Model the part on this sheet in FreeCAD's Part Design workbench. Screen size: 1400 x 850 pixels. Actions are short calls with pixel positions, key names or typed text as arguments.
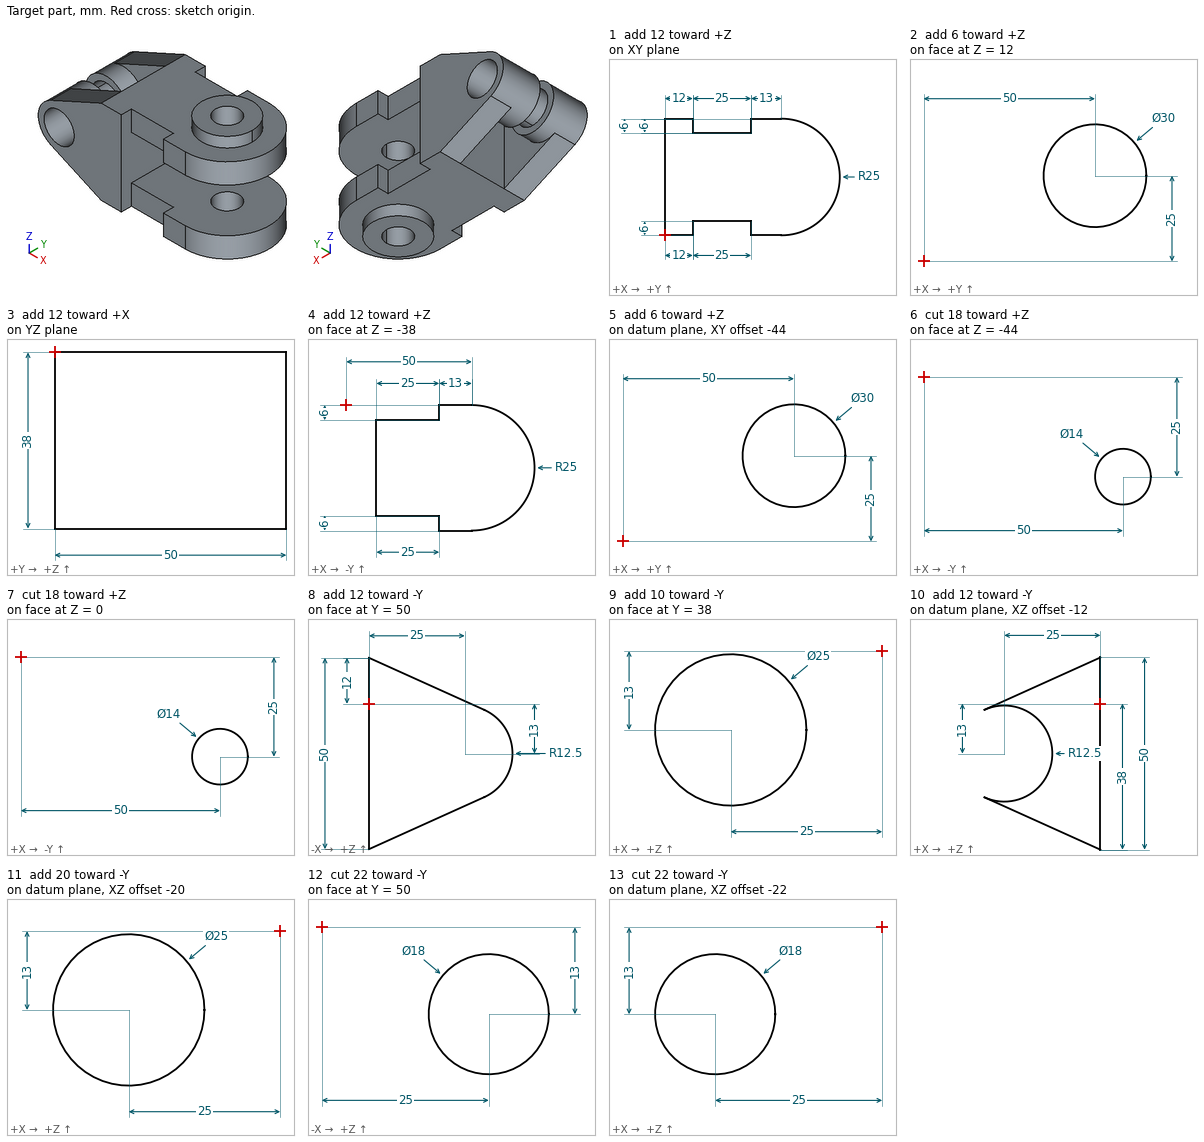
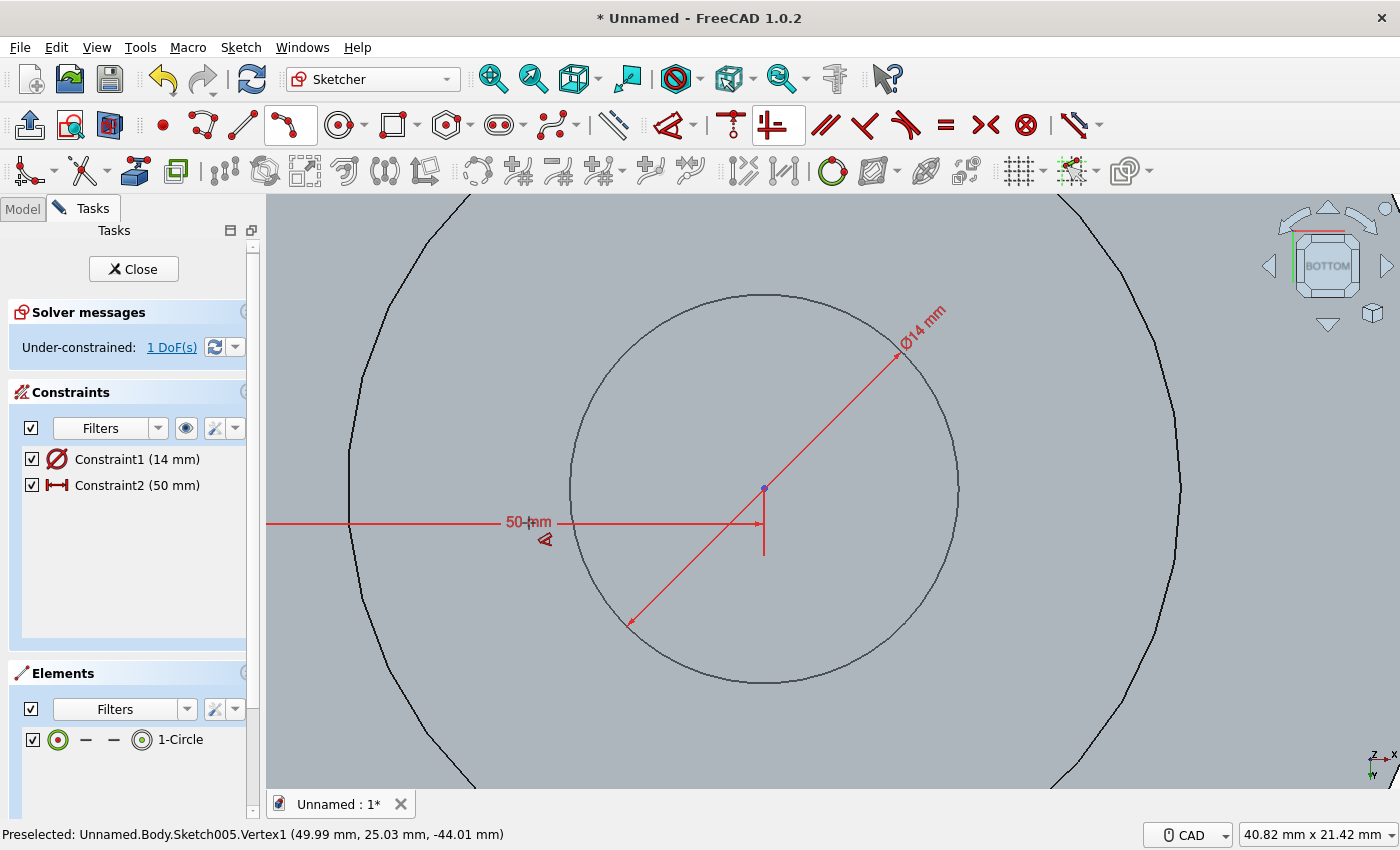
click(764, 489)
click(798, 355)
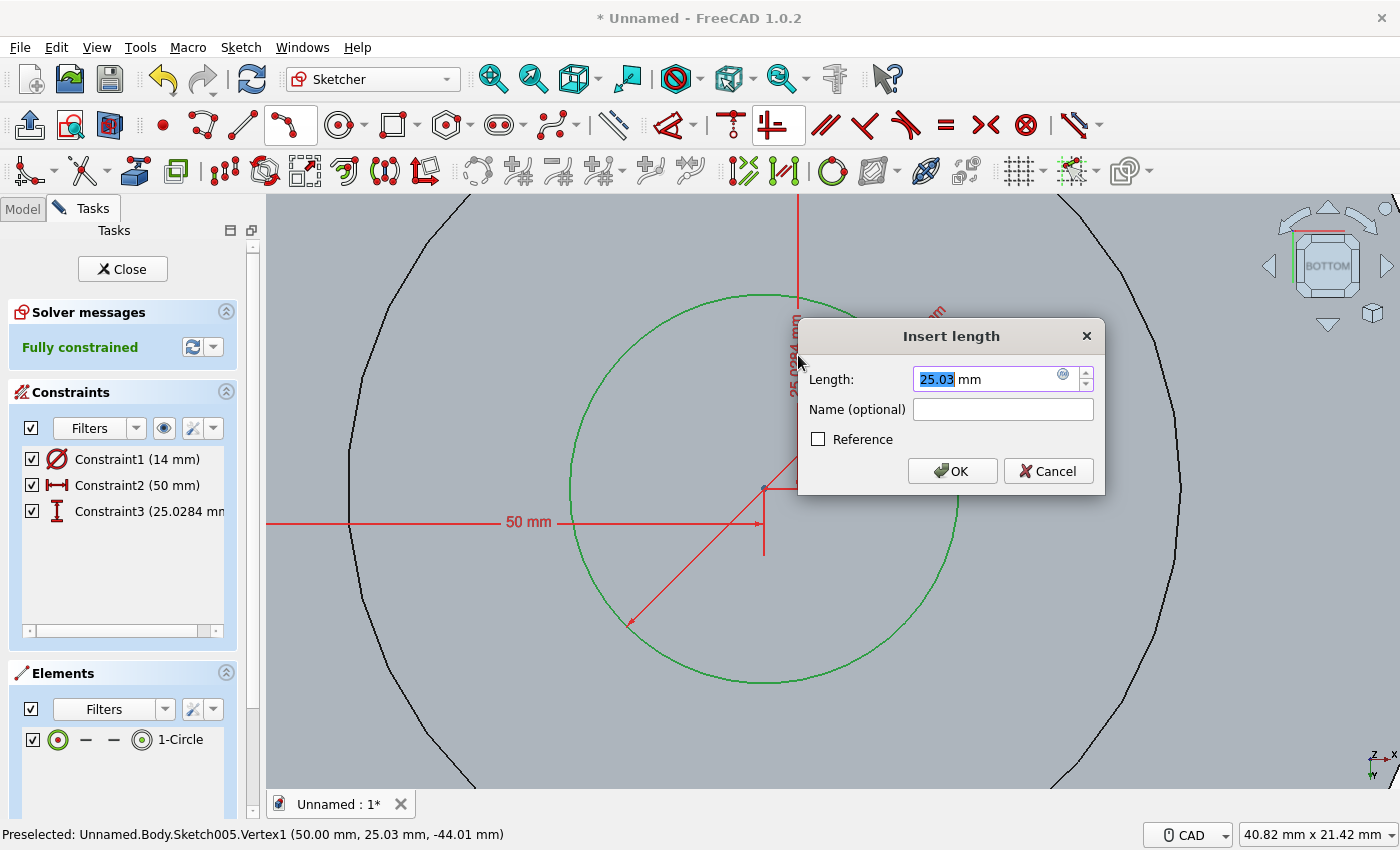
text(25)
key(Return)
key(Escape)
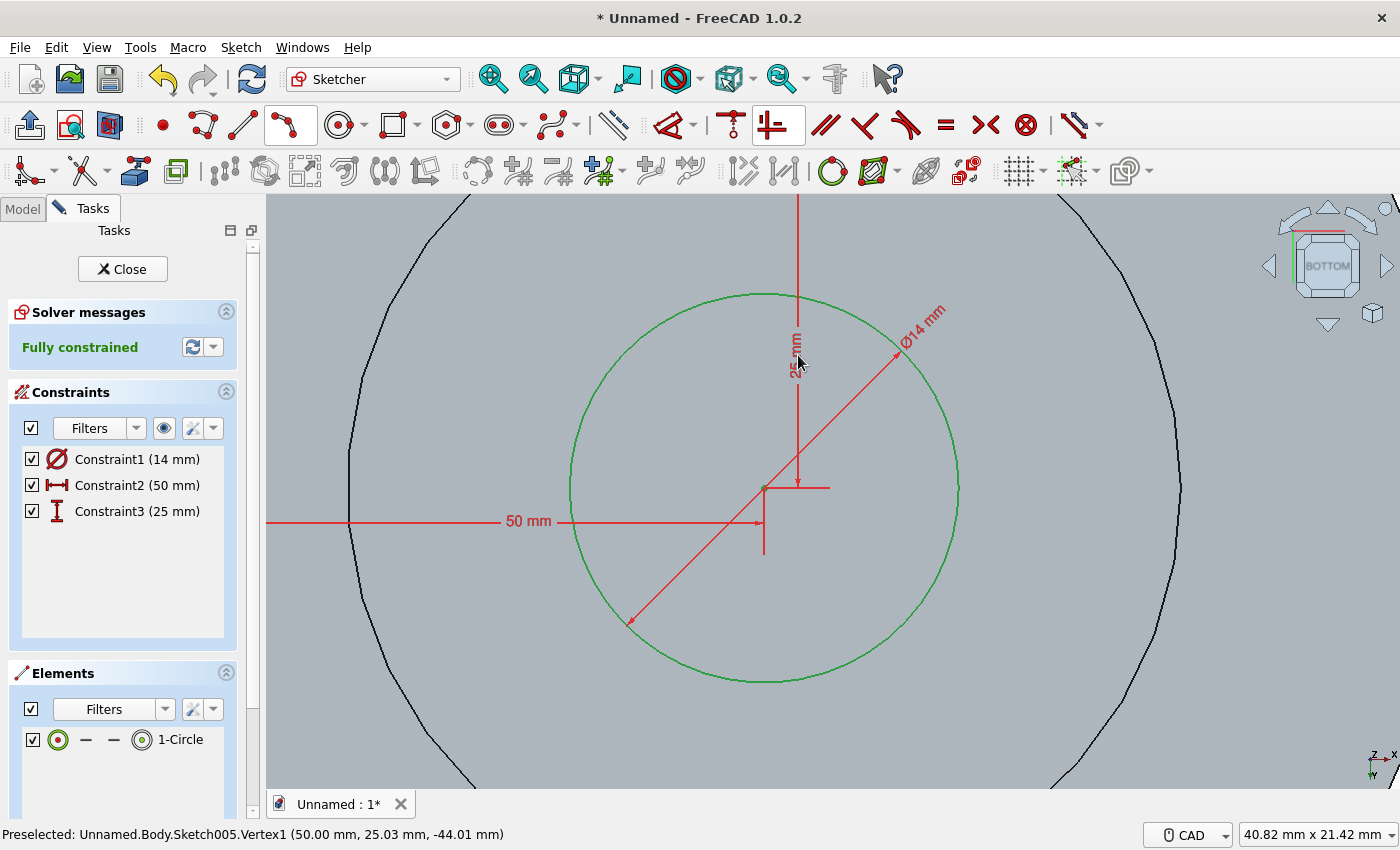
click(123, 269)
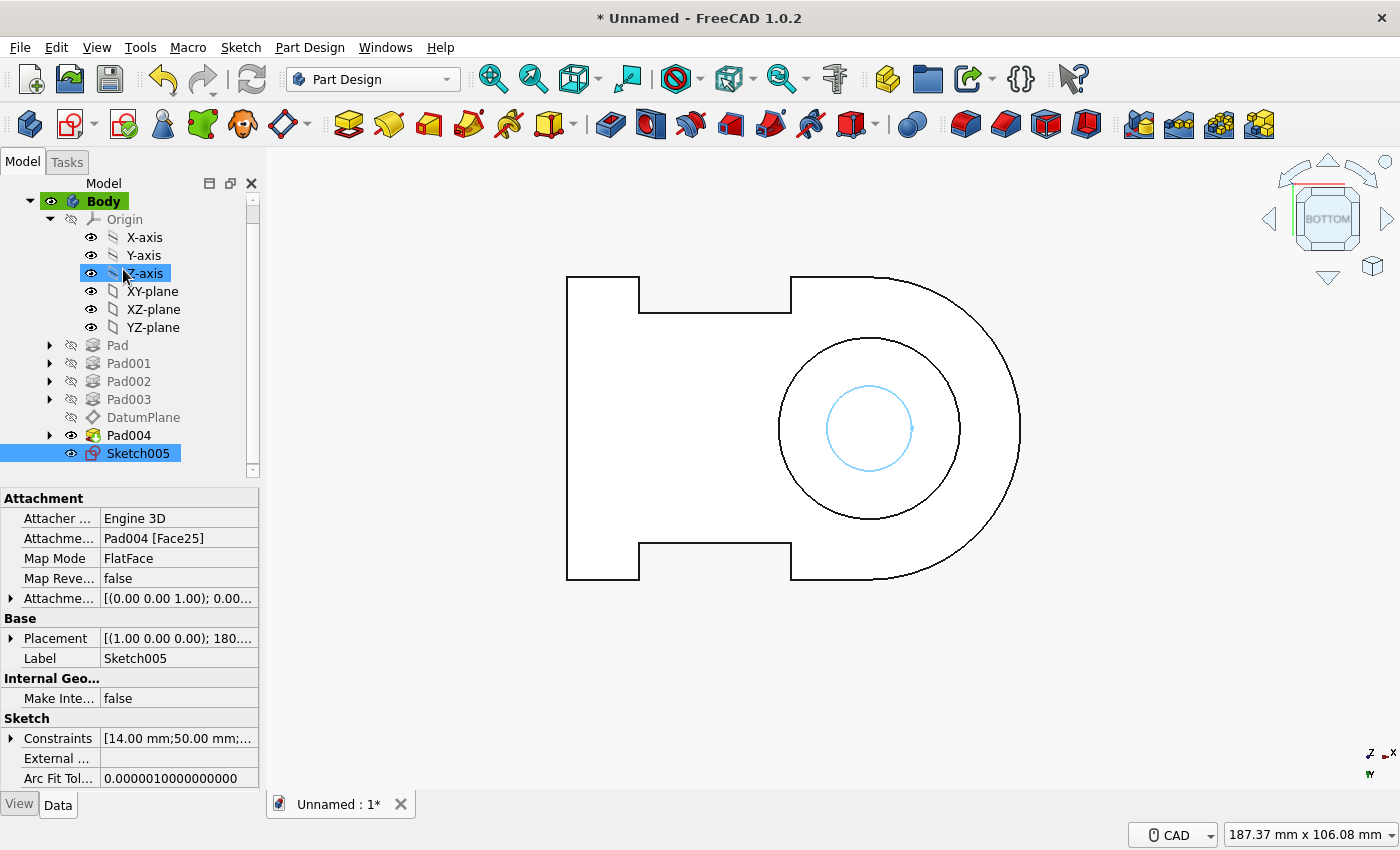
click(612, 124)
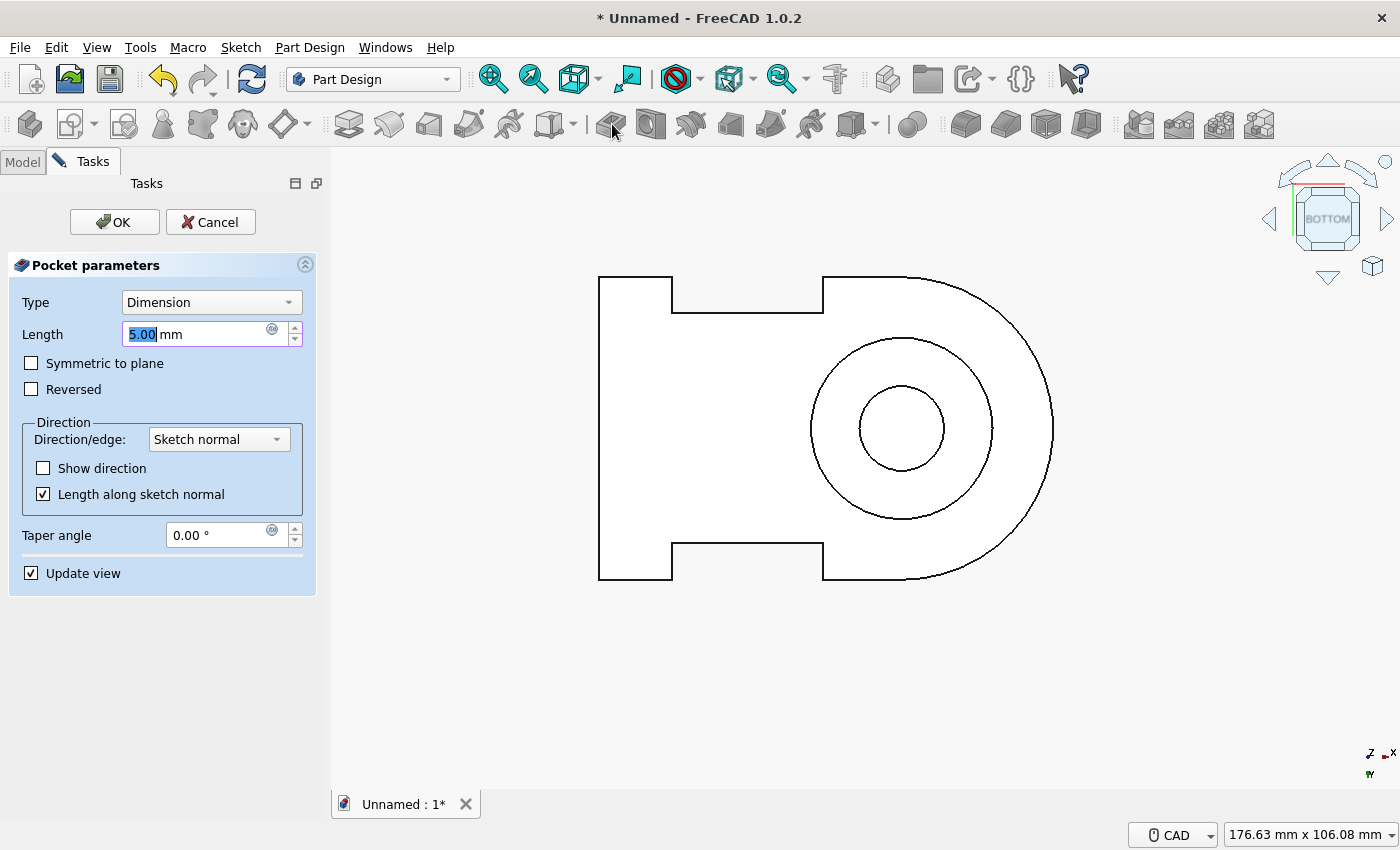
text(18)
key(Tab)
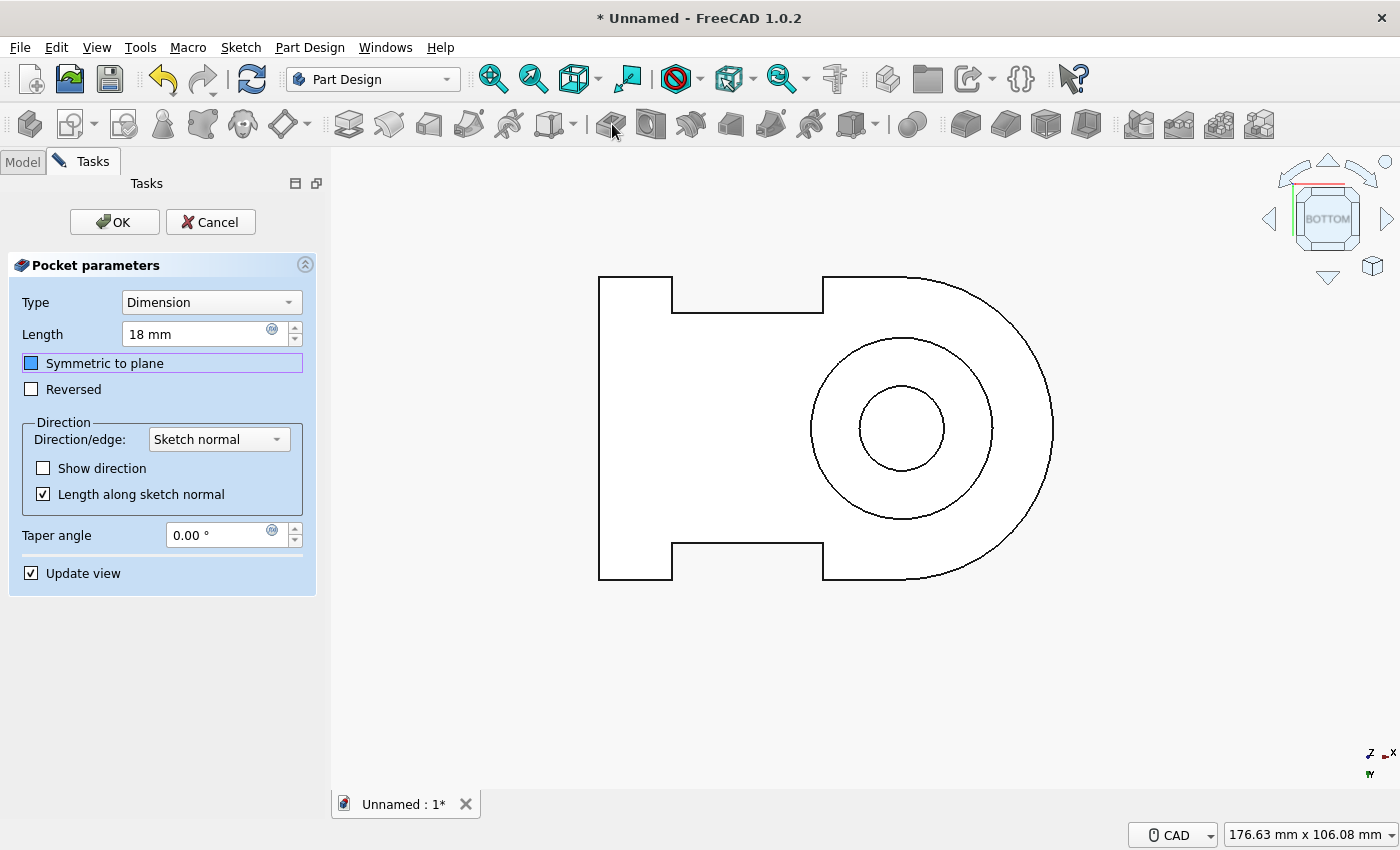
click(115, 222)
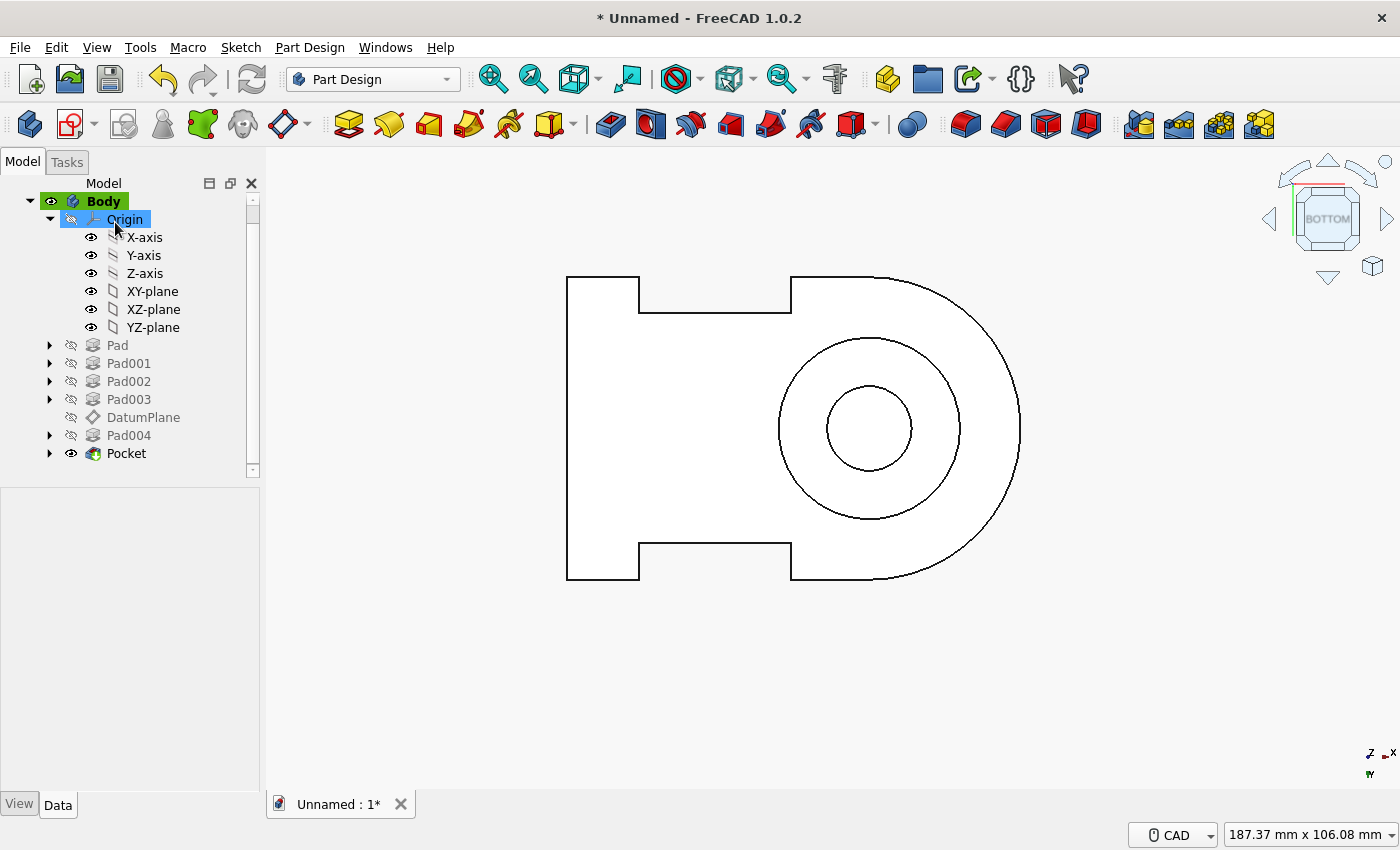
click(884, 427)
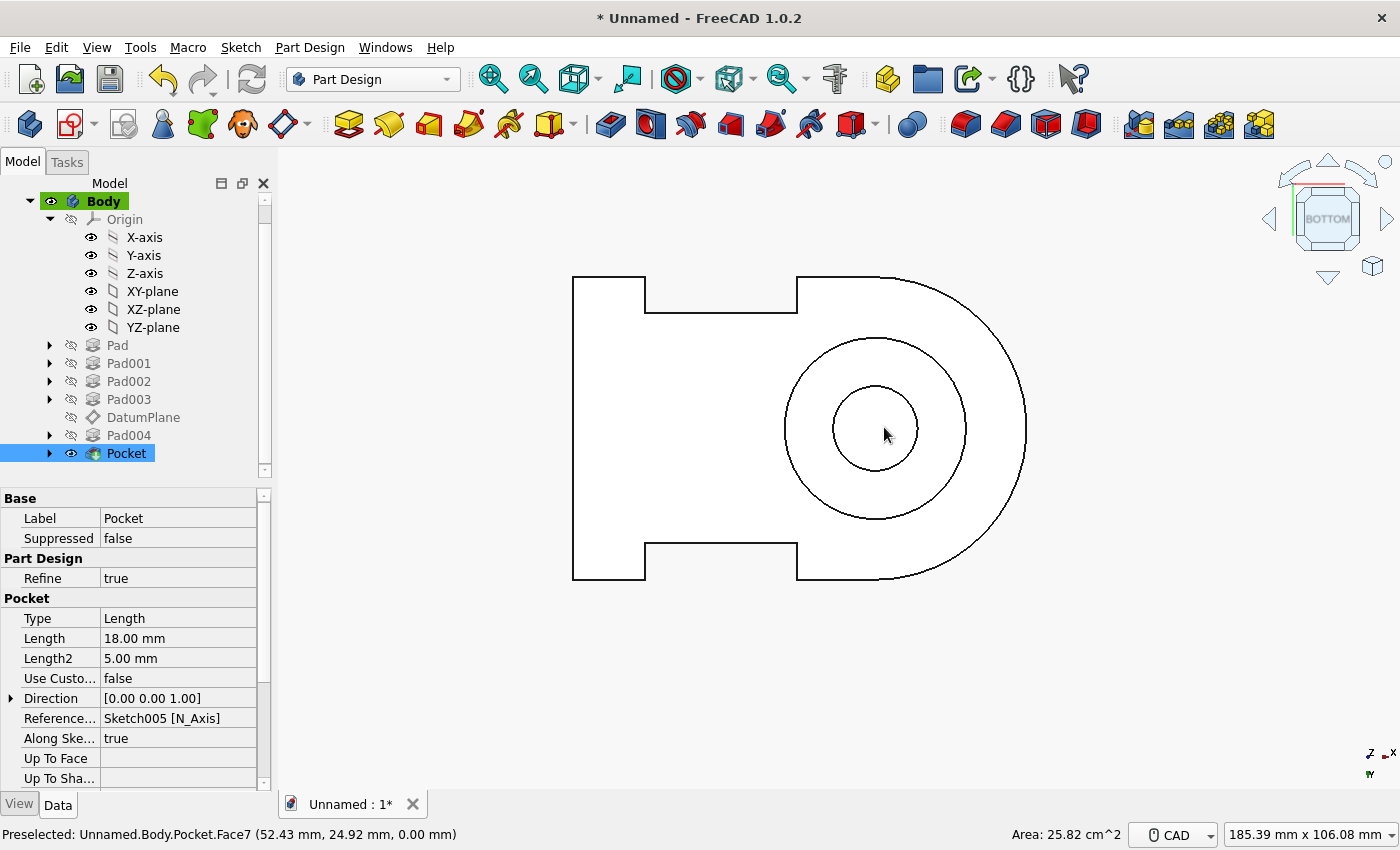
click(70, 124)